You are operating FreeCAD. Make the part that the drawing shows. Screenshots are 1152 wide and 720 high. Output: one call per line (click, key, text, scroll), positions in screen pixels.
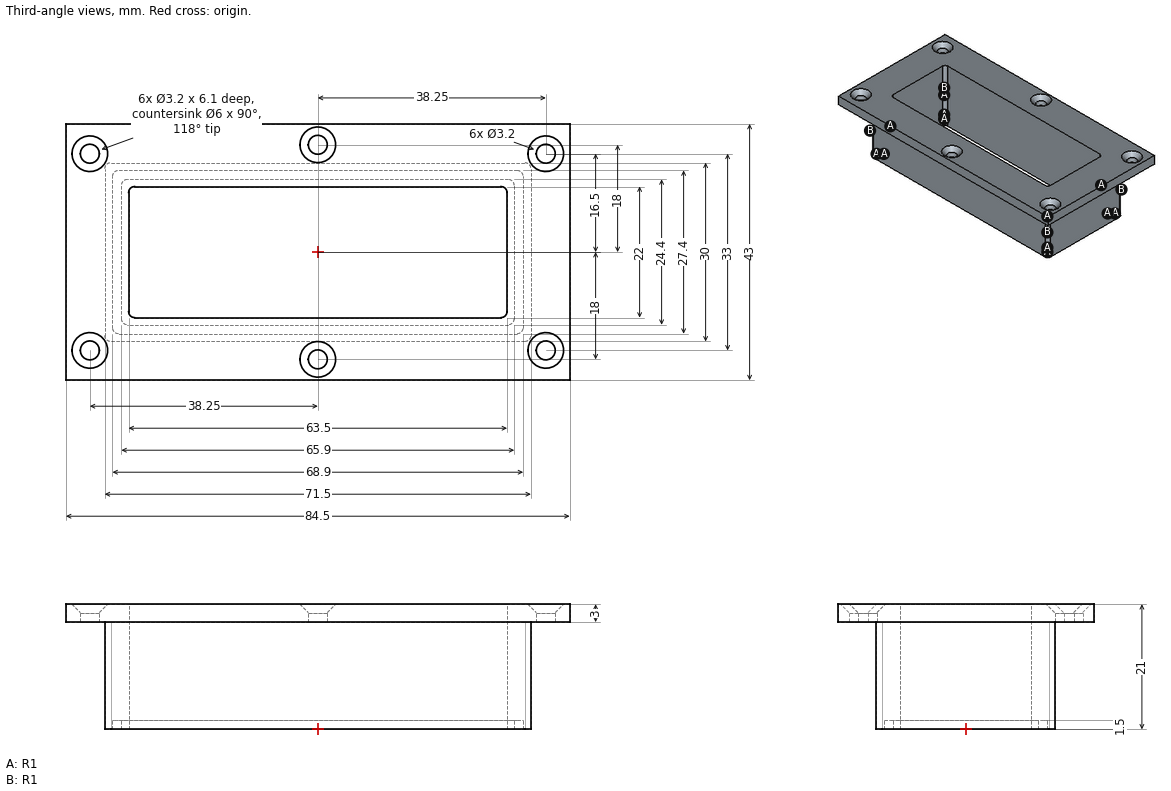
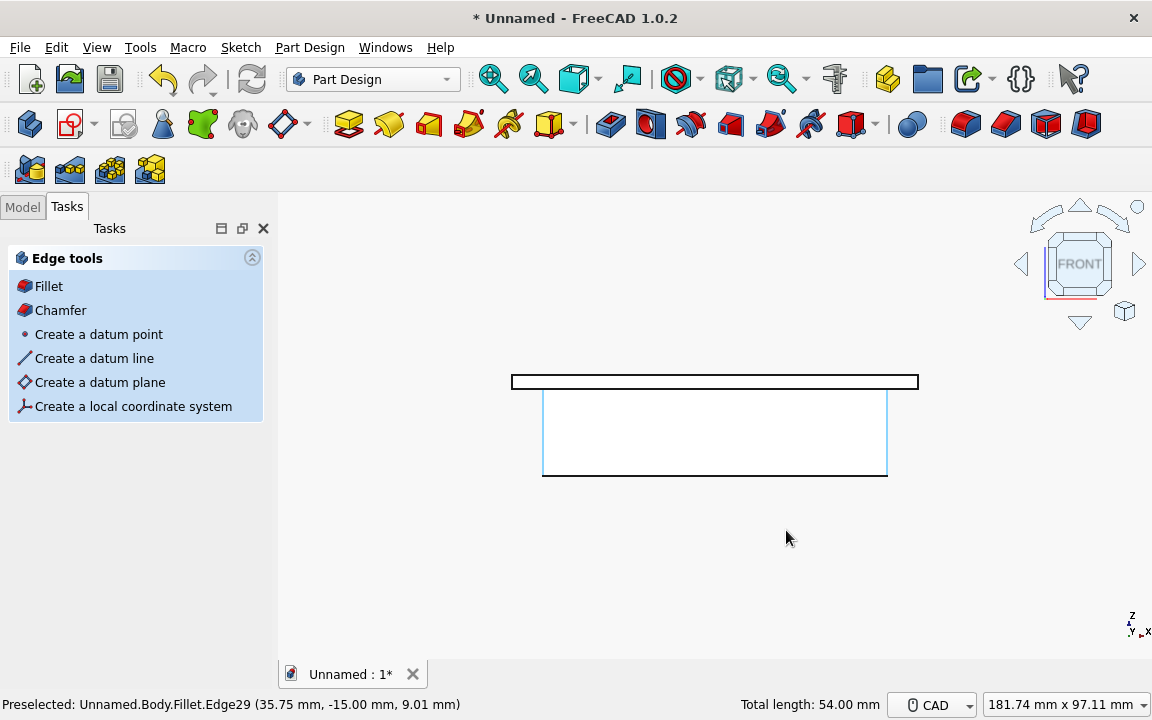
key(3)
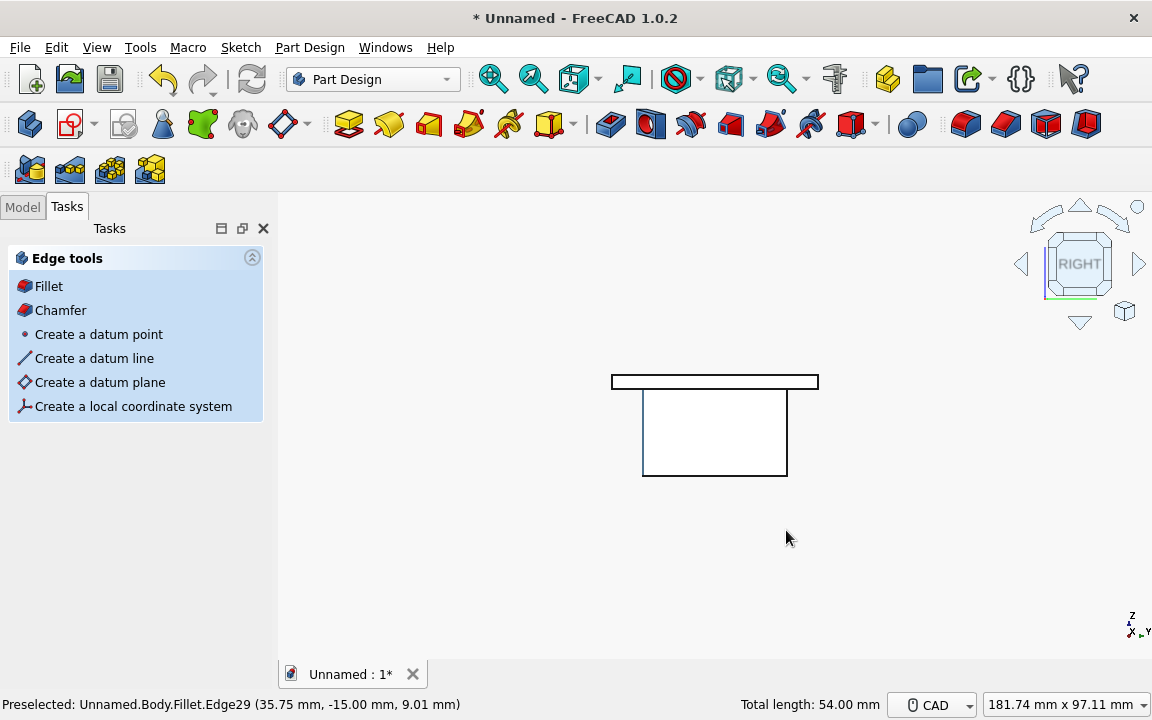
key(v)
key(f)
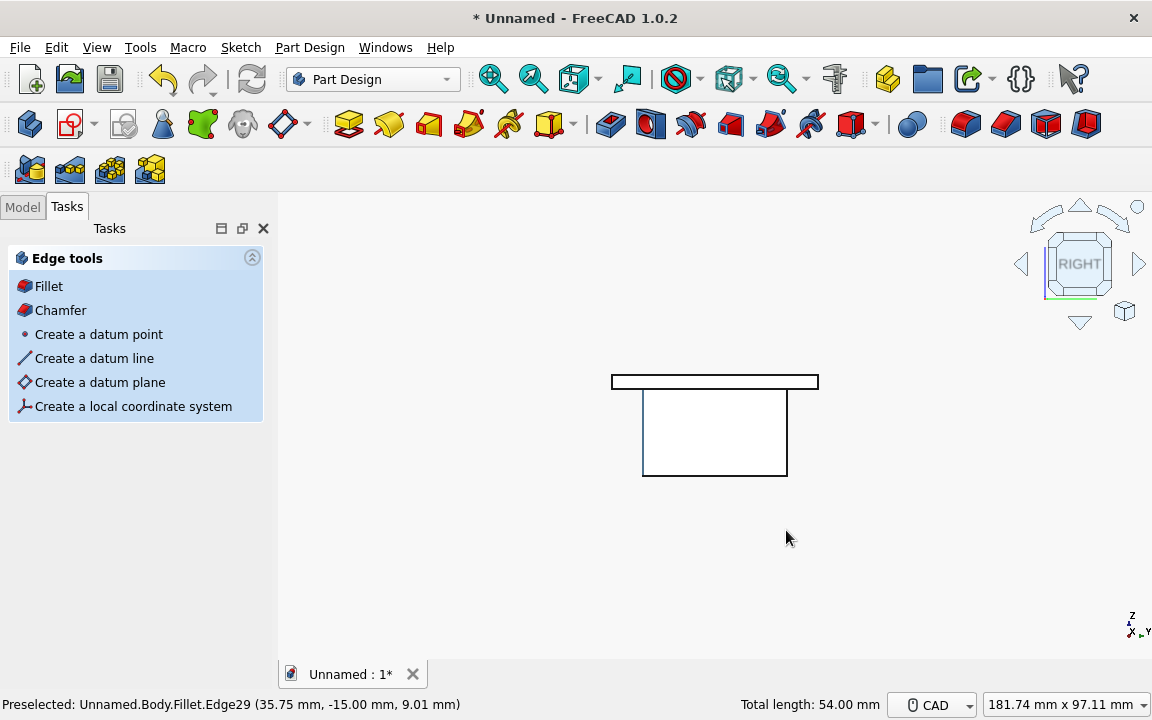
click(787, 432, ctrl)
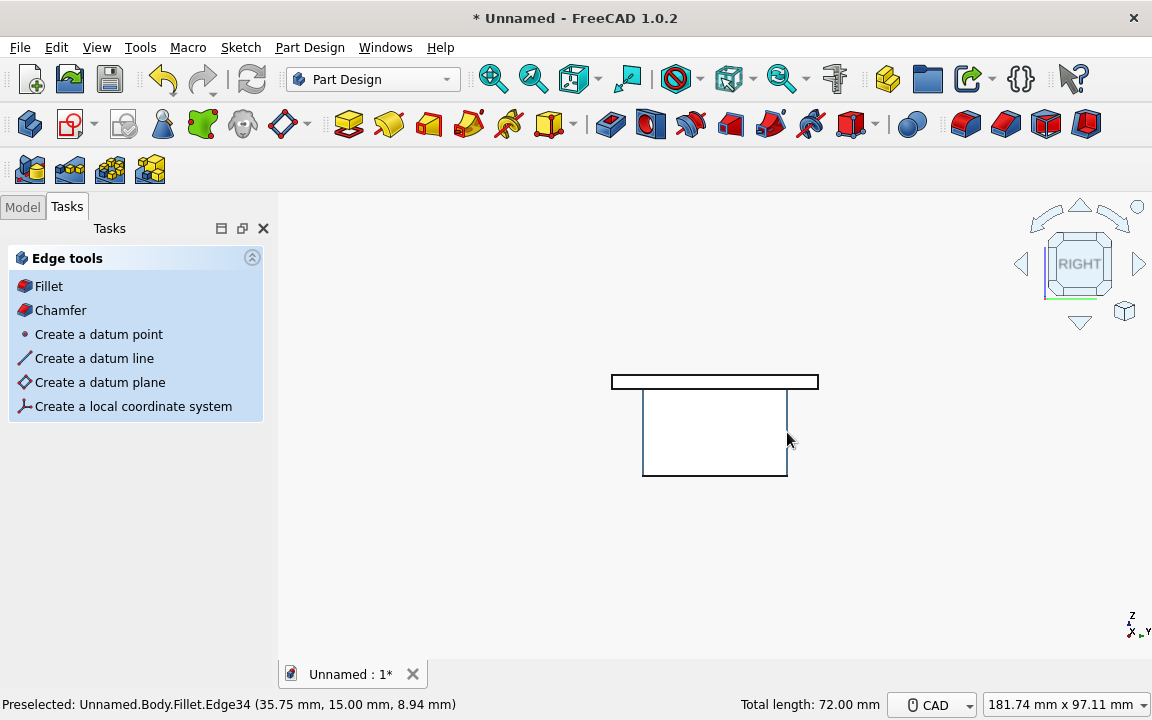
click(966, 124)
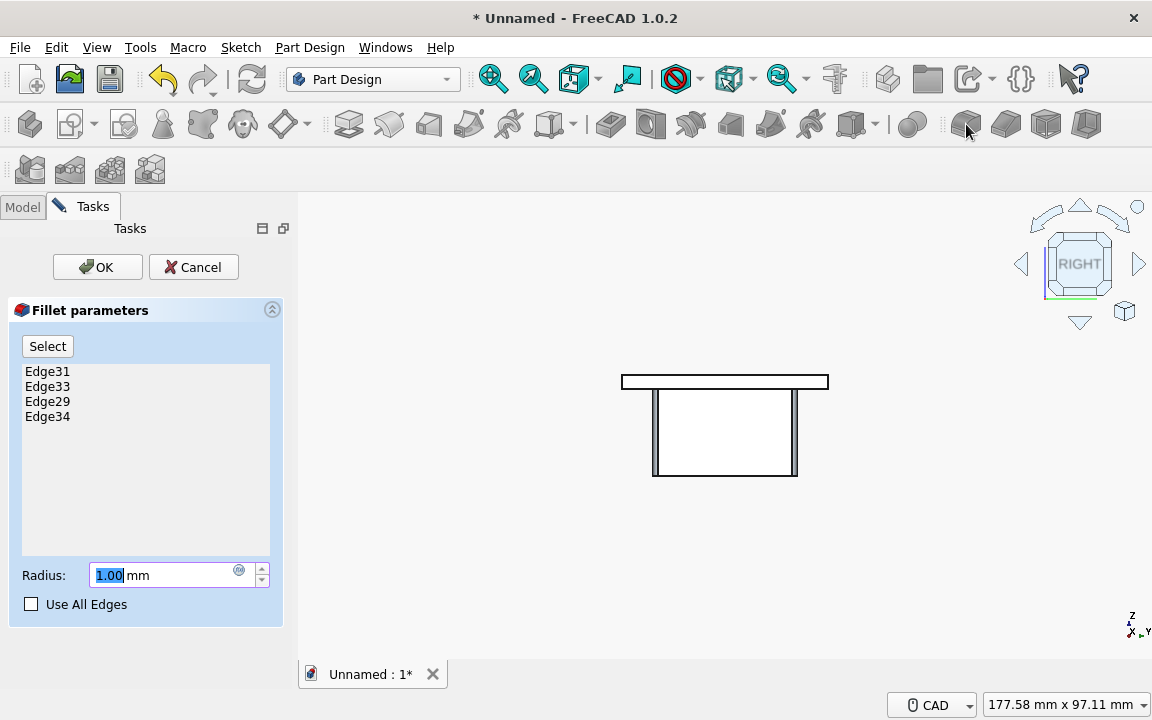
text(1)
key(Tab)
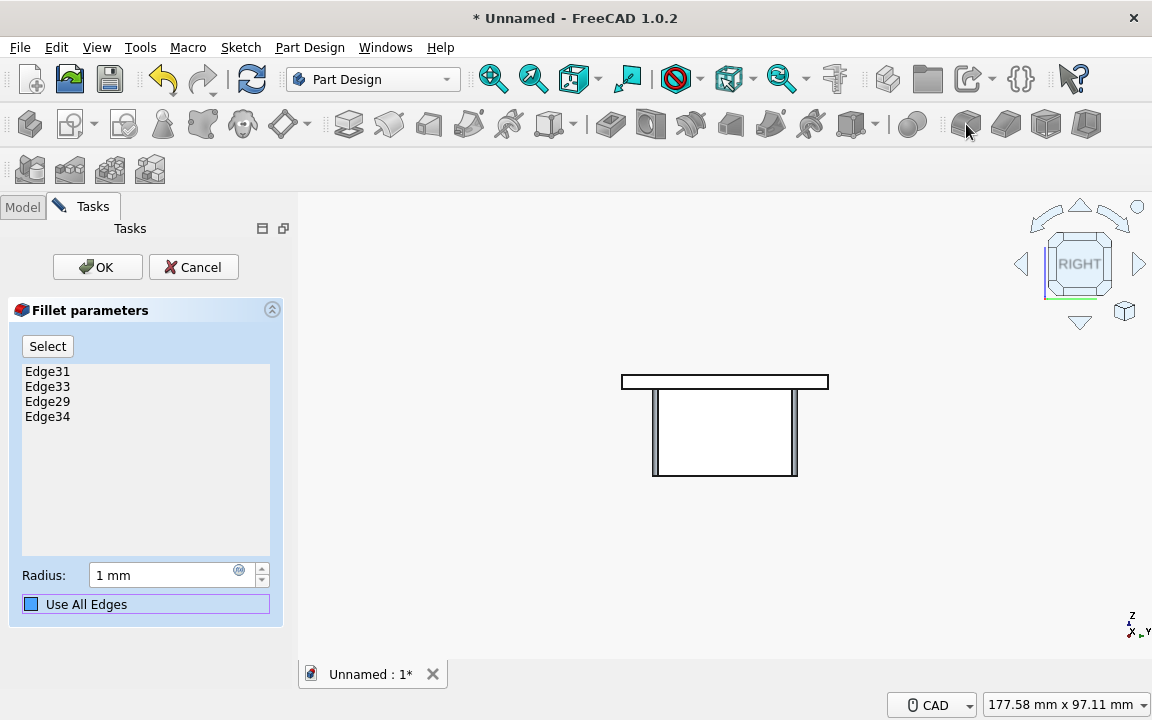
click(98, 267)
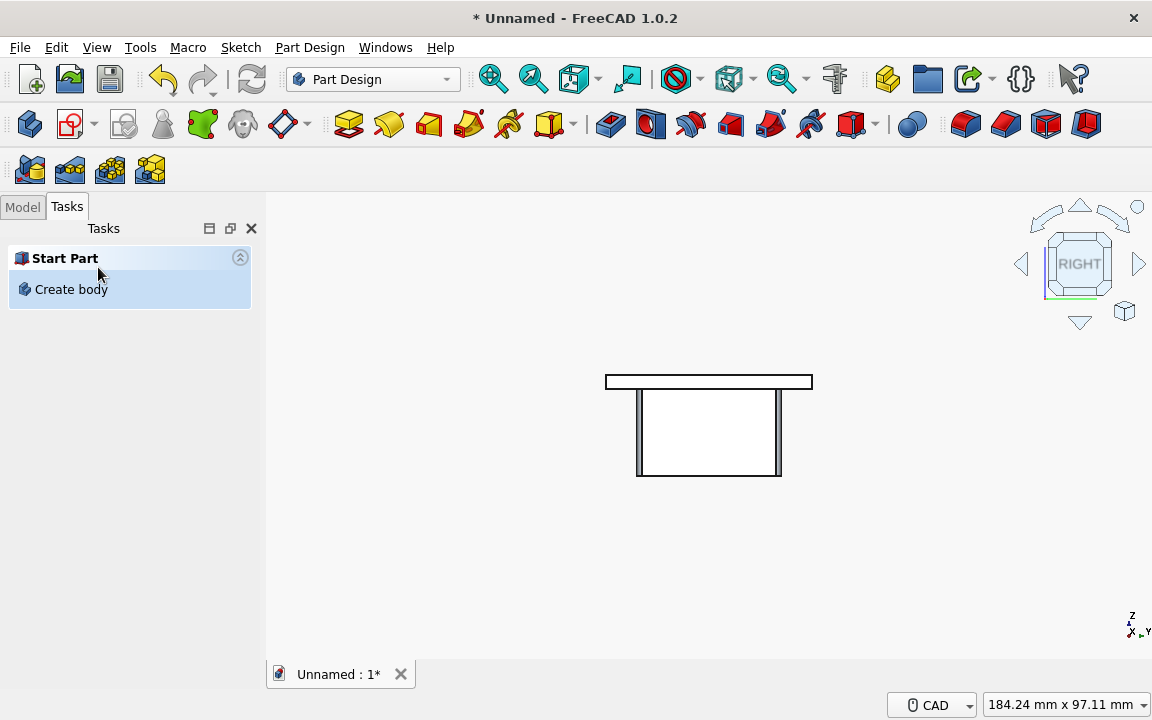
key(0)